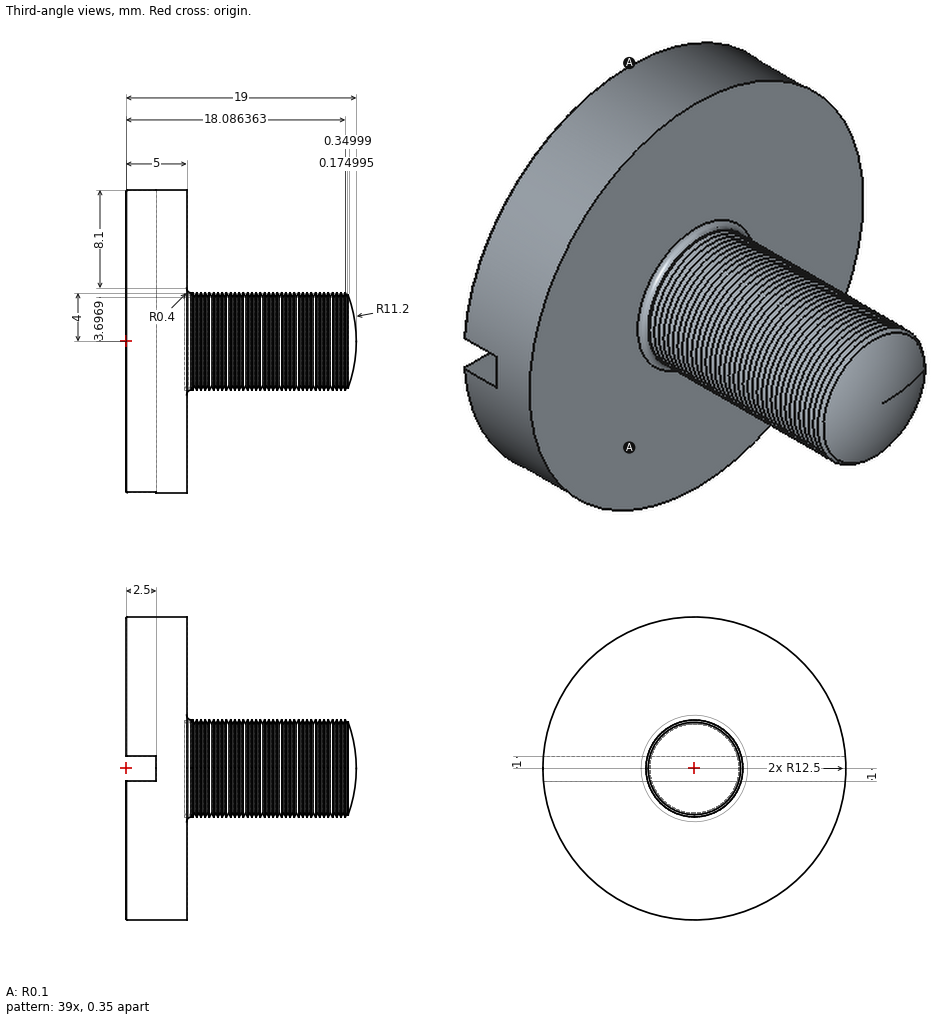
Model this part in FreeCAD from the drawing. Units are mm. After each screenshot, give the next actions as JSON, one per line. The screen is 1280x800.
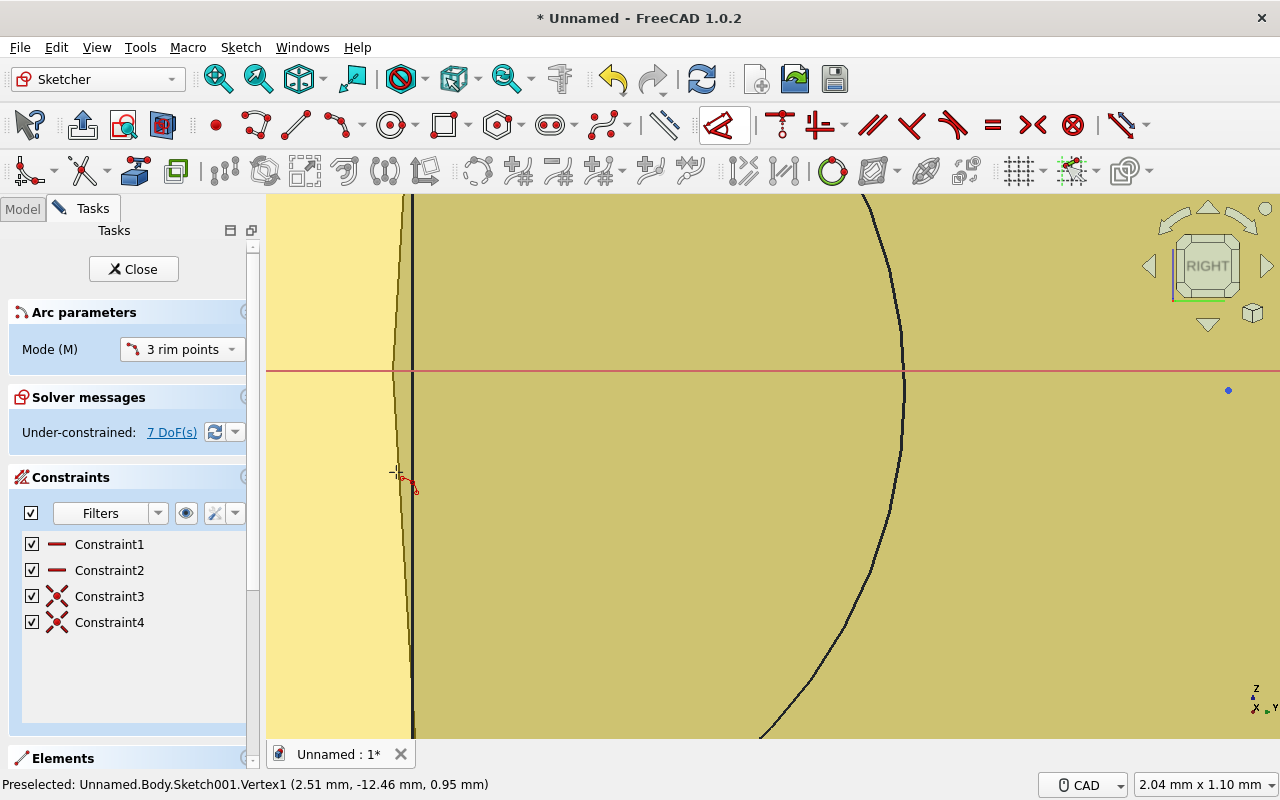
{"action": "left_click", "coordinate": [394, 470]}
{"action": "key", "text": "Escape"}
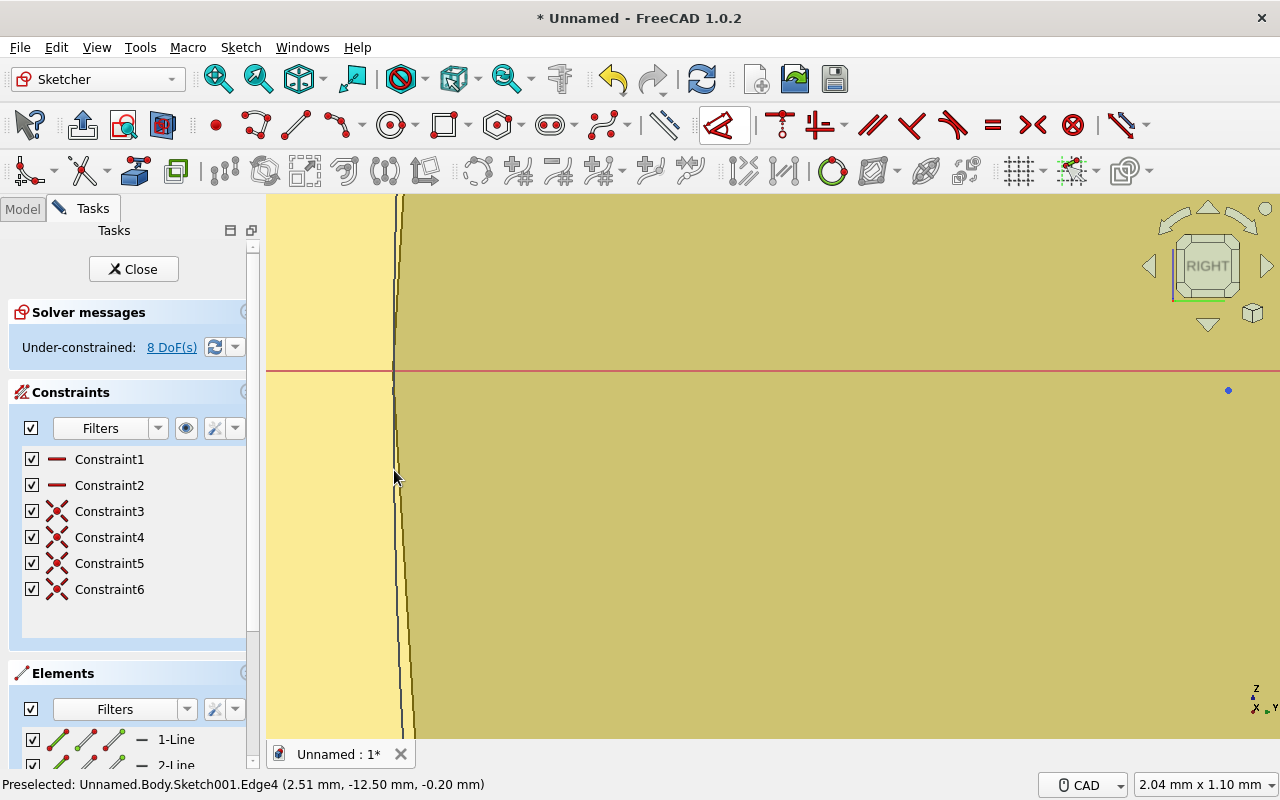
{"action": "scroll", "coordinate": [395, 472], "scroll_direction": "down", "scroll_amount": 15}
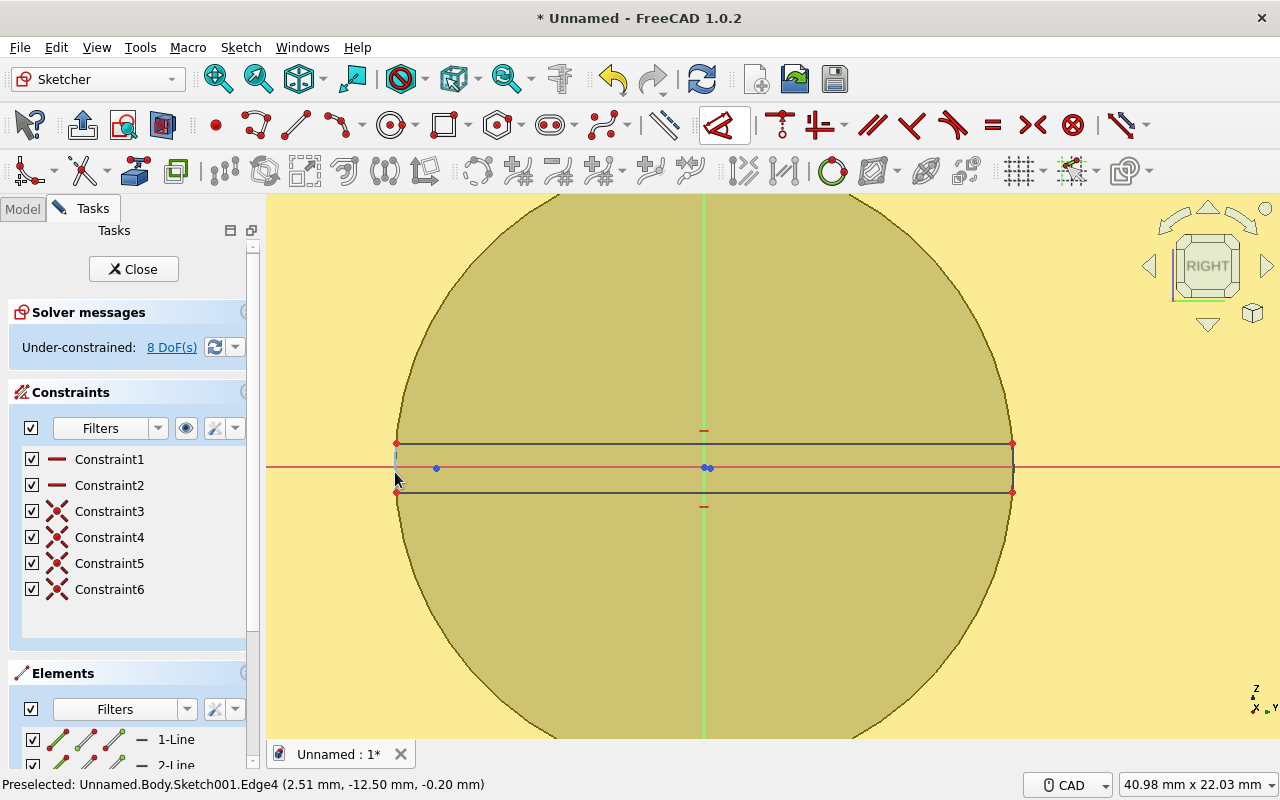
{"action": "scroll", "coordinate": [1013, 478], "scroll_direction": "up", "scroll_amount": 2}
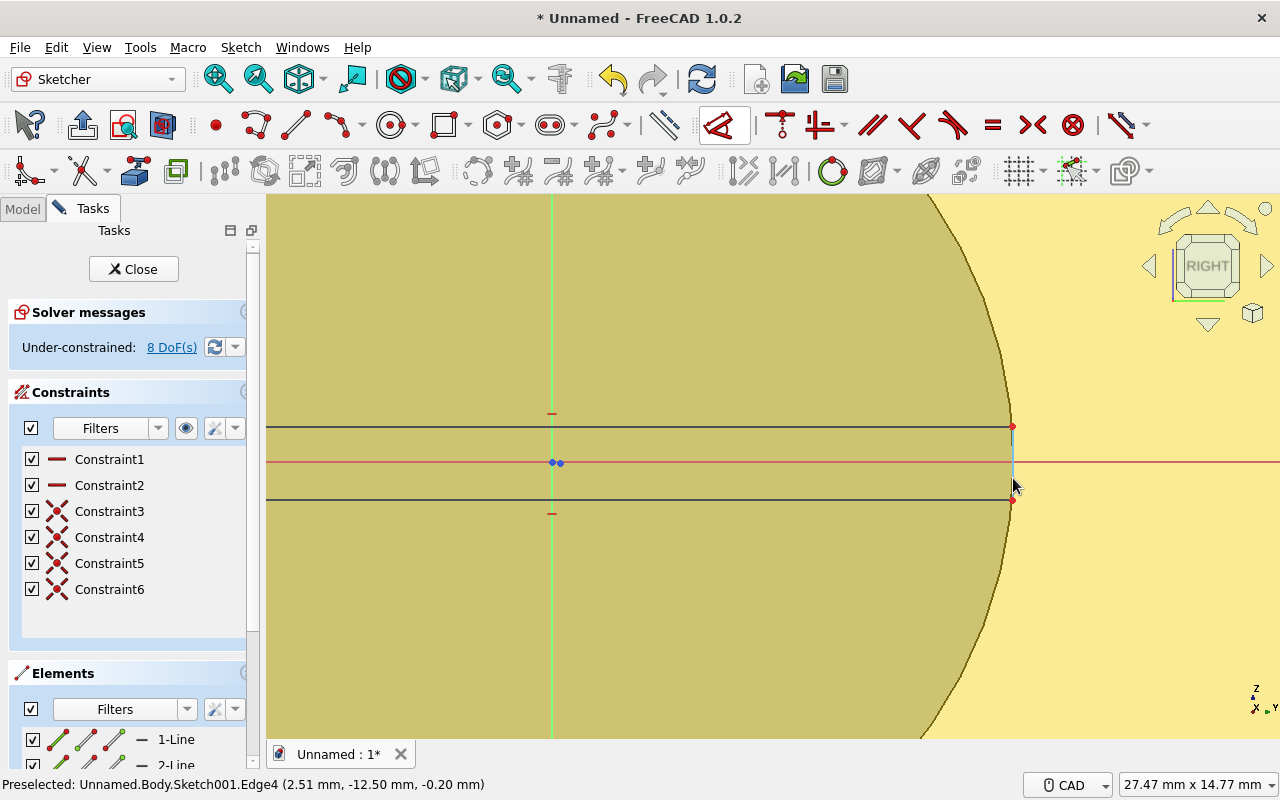
{"action": "left_click", "coordinate": [1013, 478]}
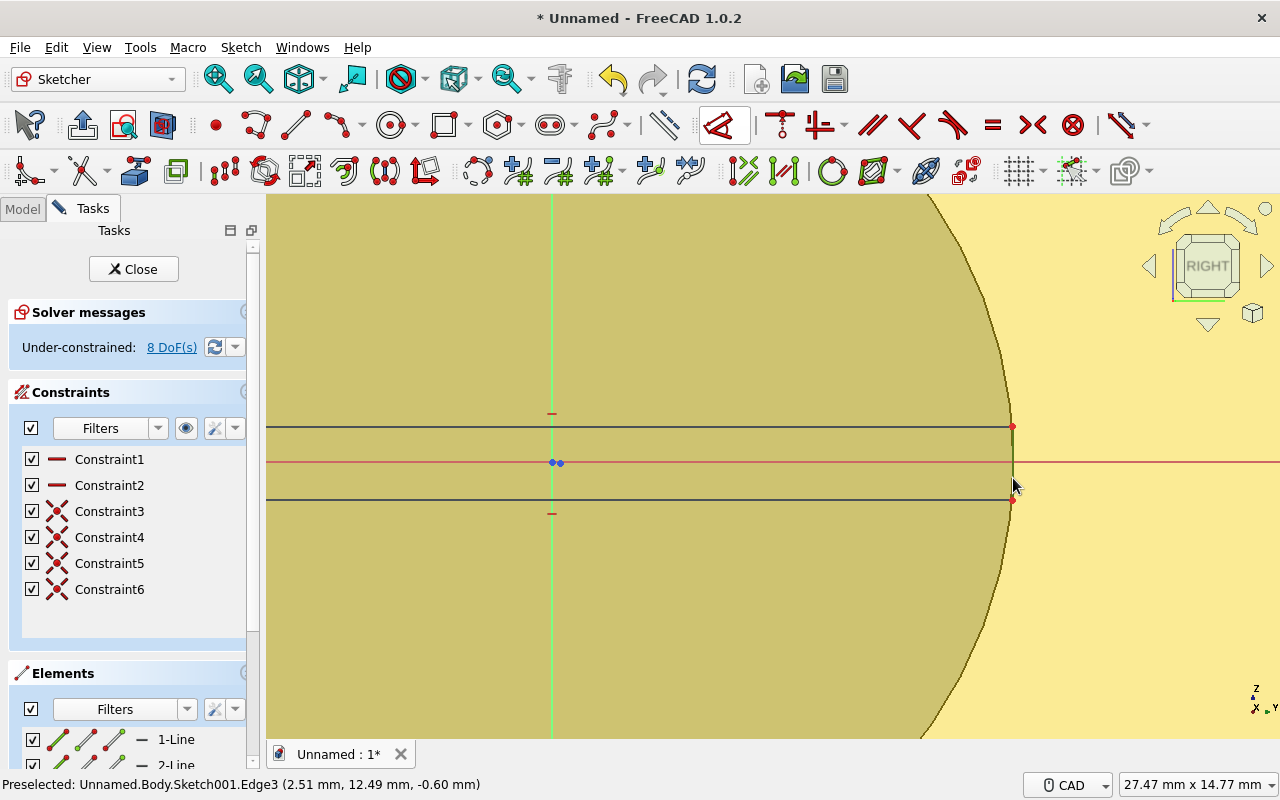
{"action": "scroll", "coordinate": [1014, 476], "scroll_direction": "down", "scroll_amount": 2}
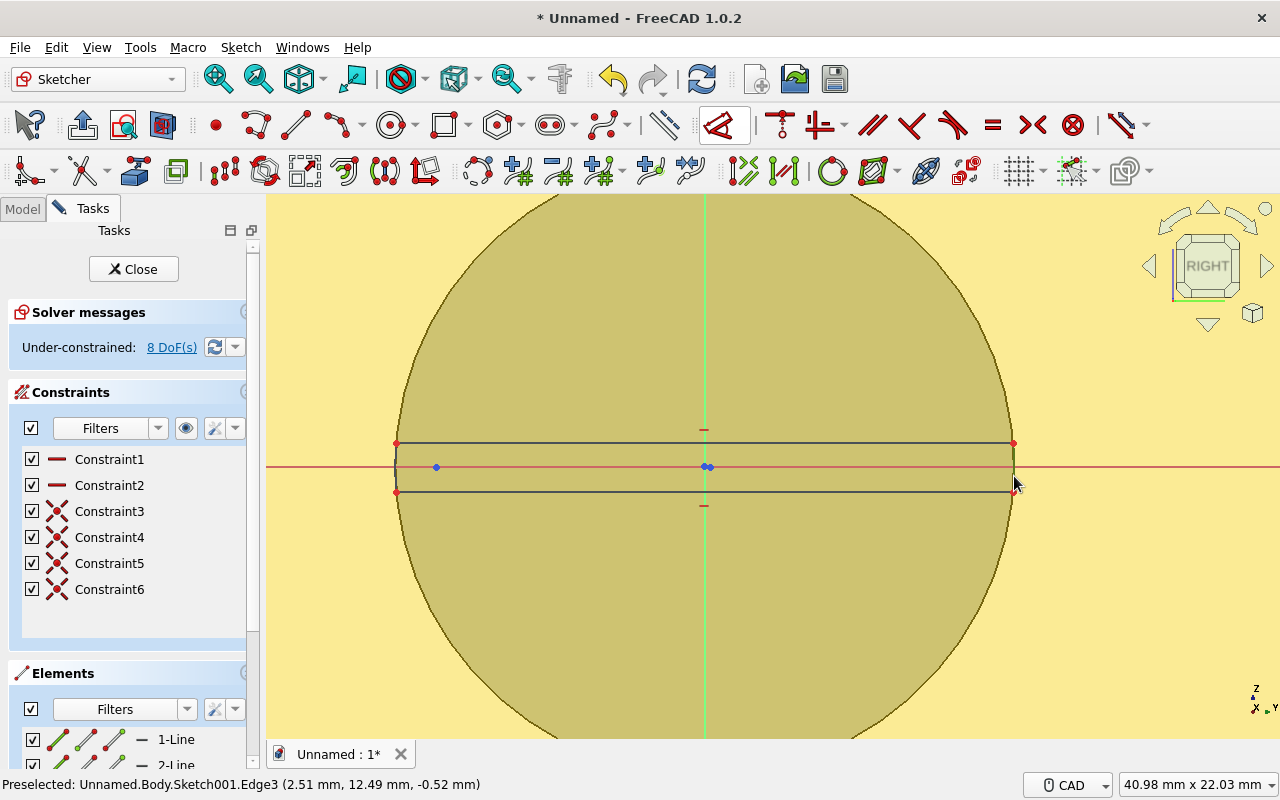
{"action": "scroll", "coordinate": [396, 458], "scroll_direction": "up", "scroll_amount": 3}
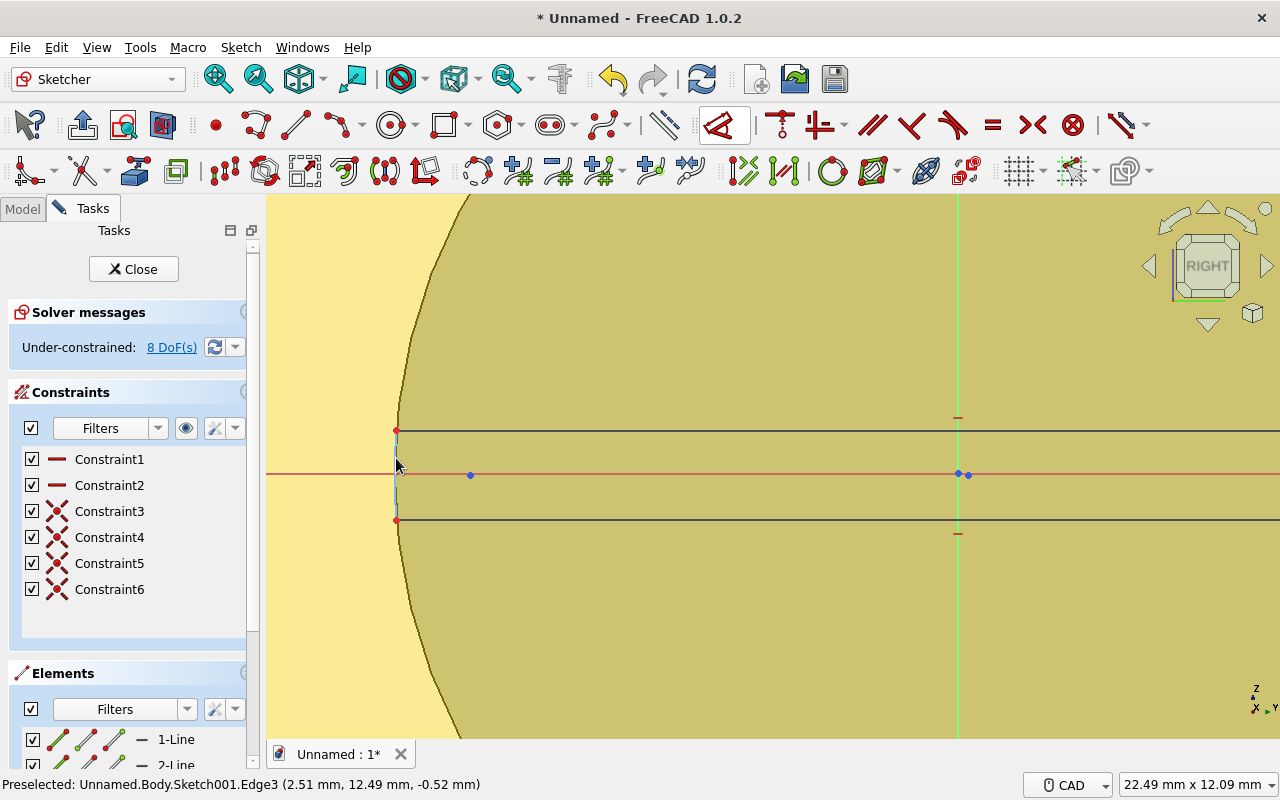
{"action": "left_click", "coordinate": [395, 458]}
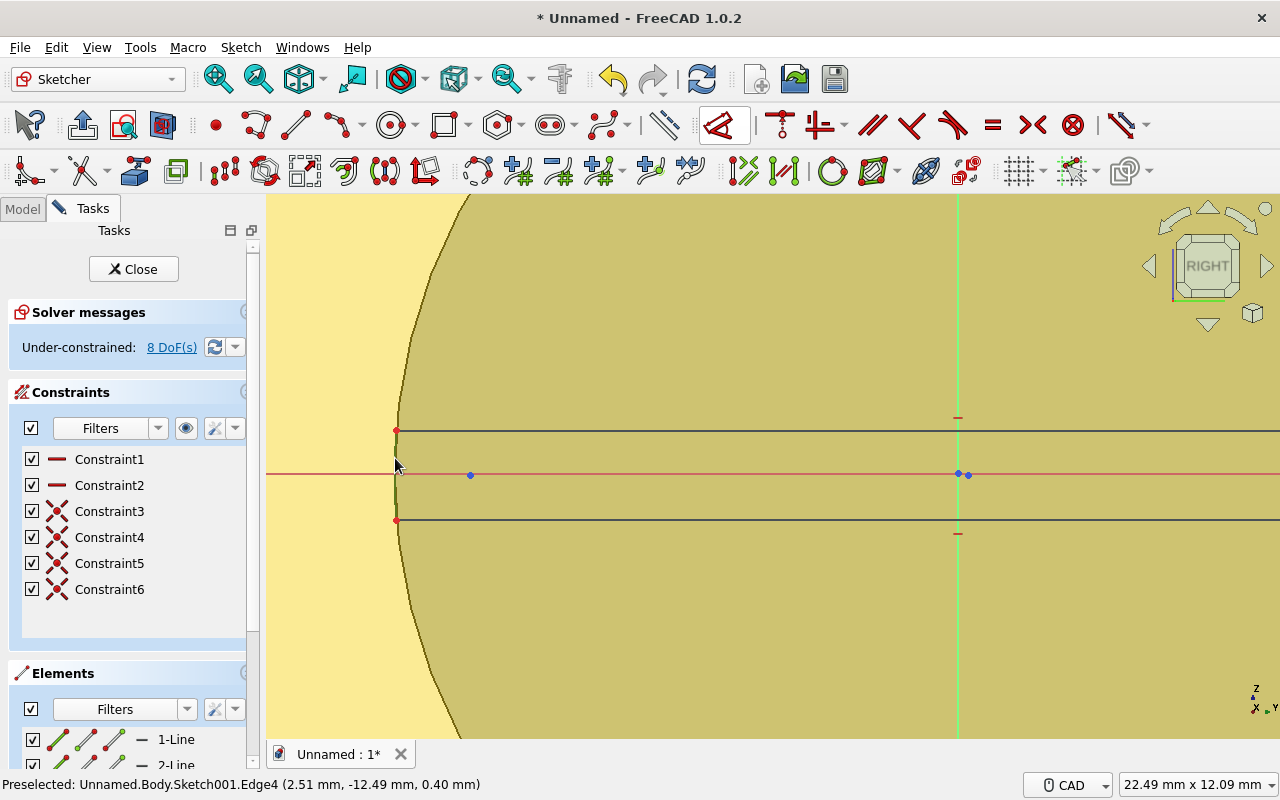
{"action": "left_click", "coordinate": [780, 126]}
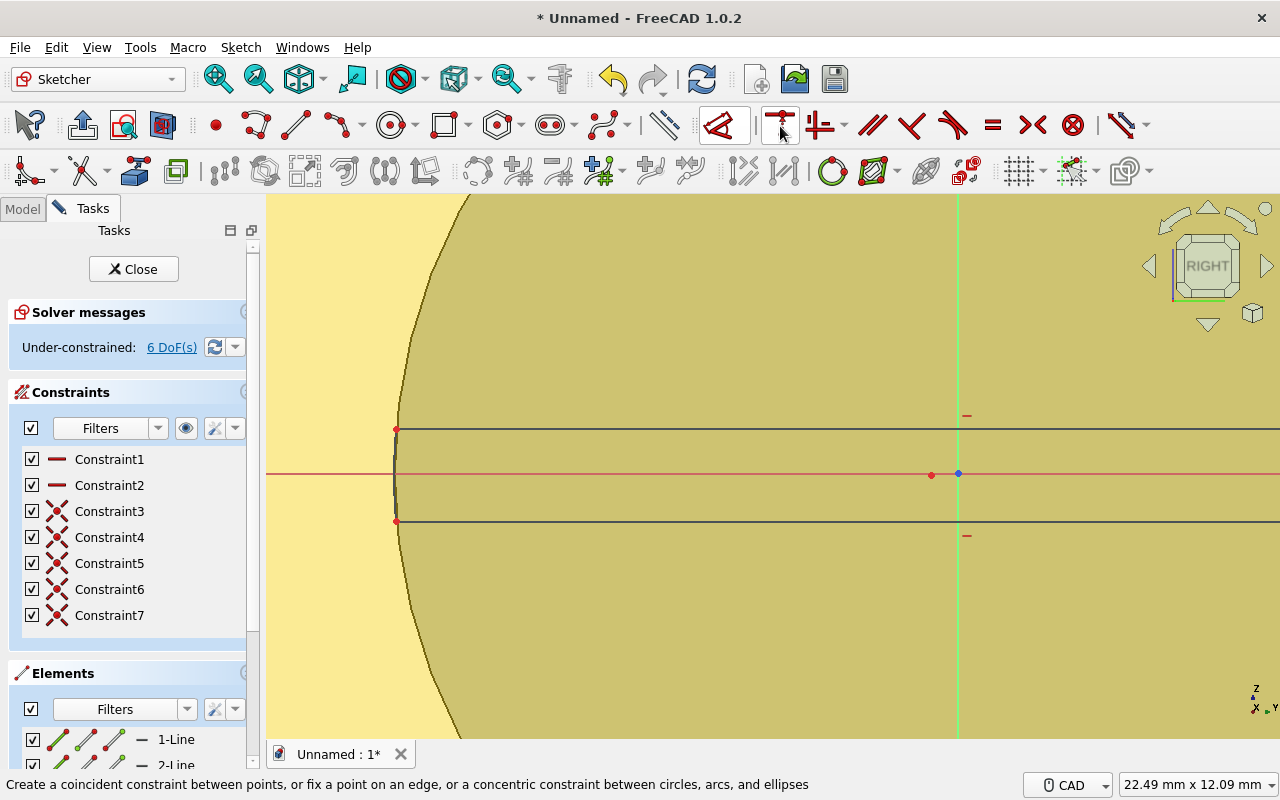
{"action": "left_click_drag", "start_coordinate": [921, 464], "coordinate": [968, 485]}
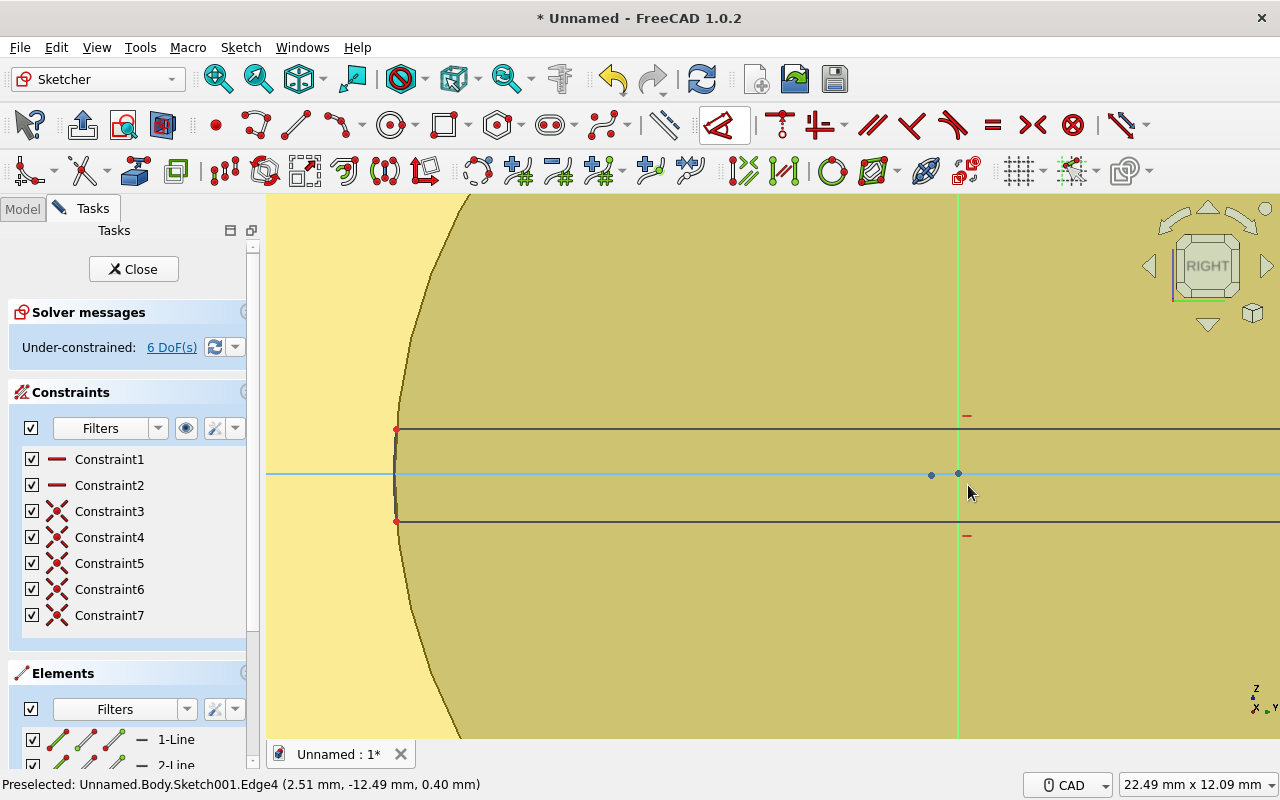
{"action": "left_click", "coordinate": [780, 126]}